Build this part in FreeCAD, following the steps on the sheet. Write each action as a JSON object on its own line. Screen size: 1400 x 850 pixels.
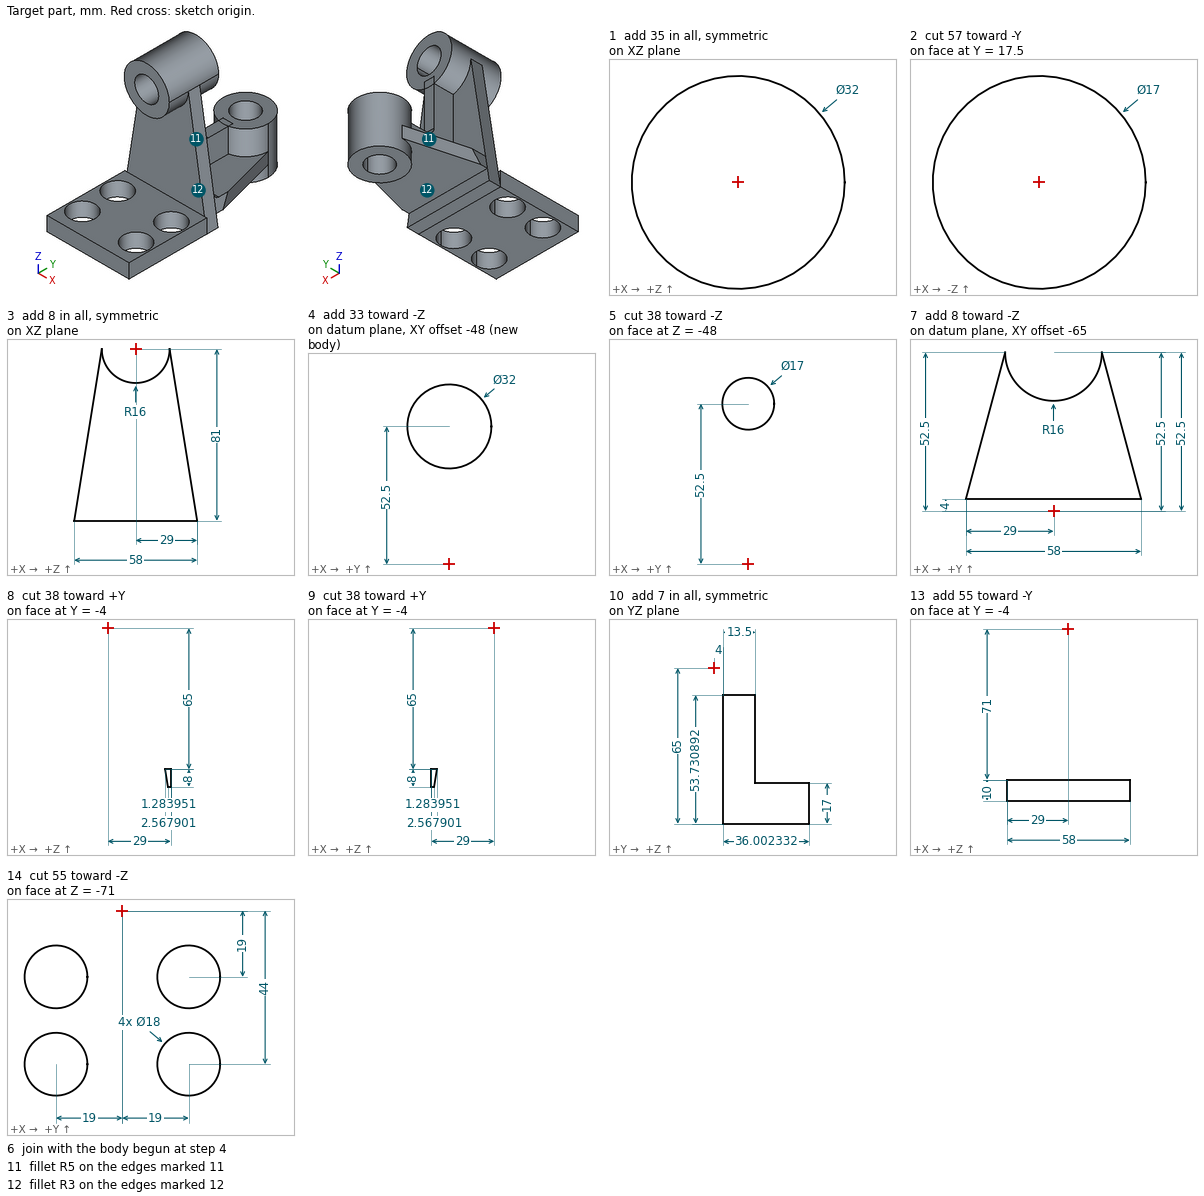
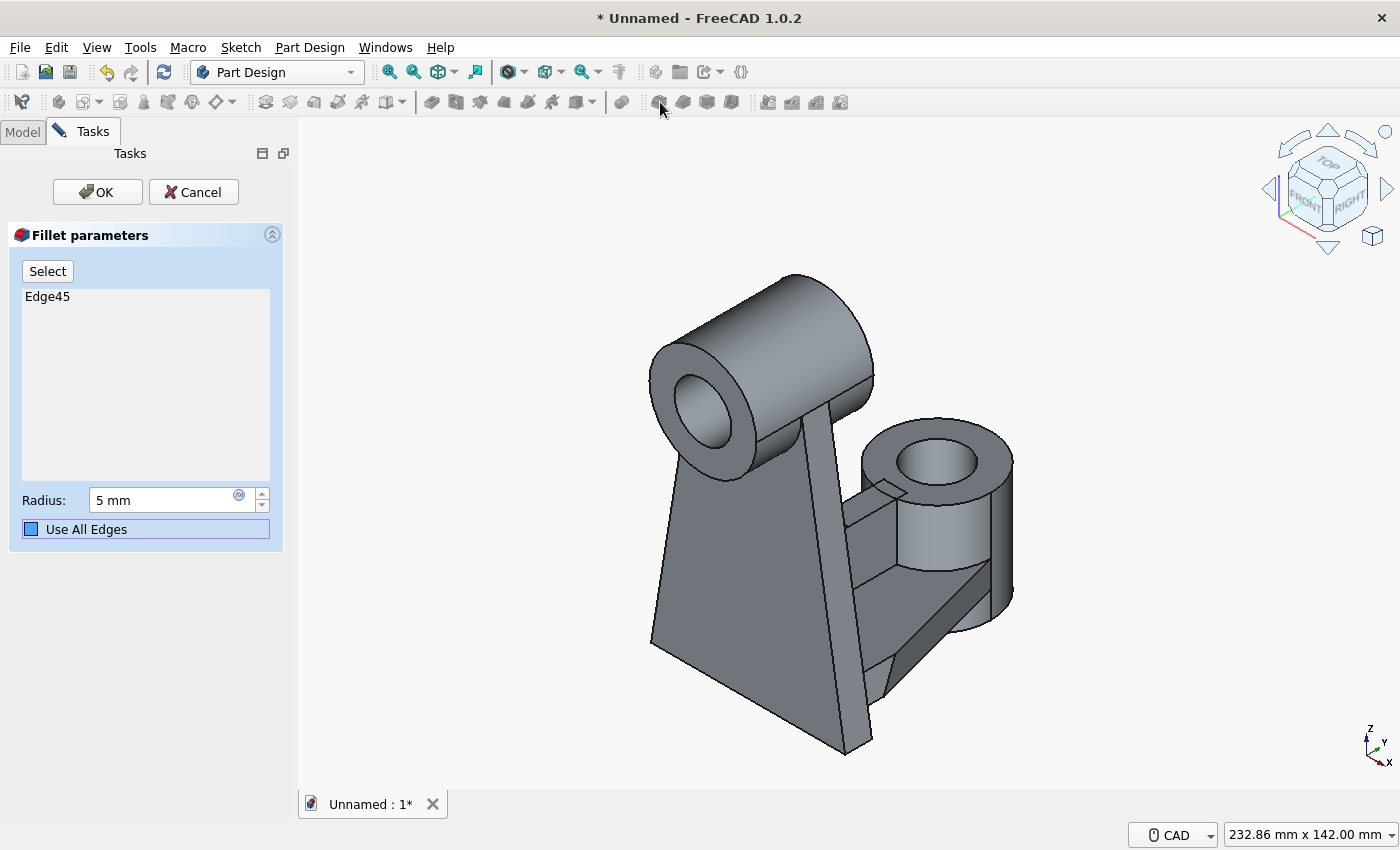
{"action": "left_click", "coordinate": [98, 192]}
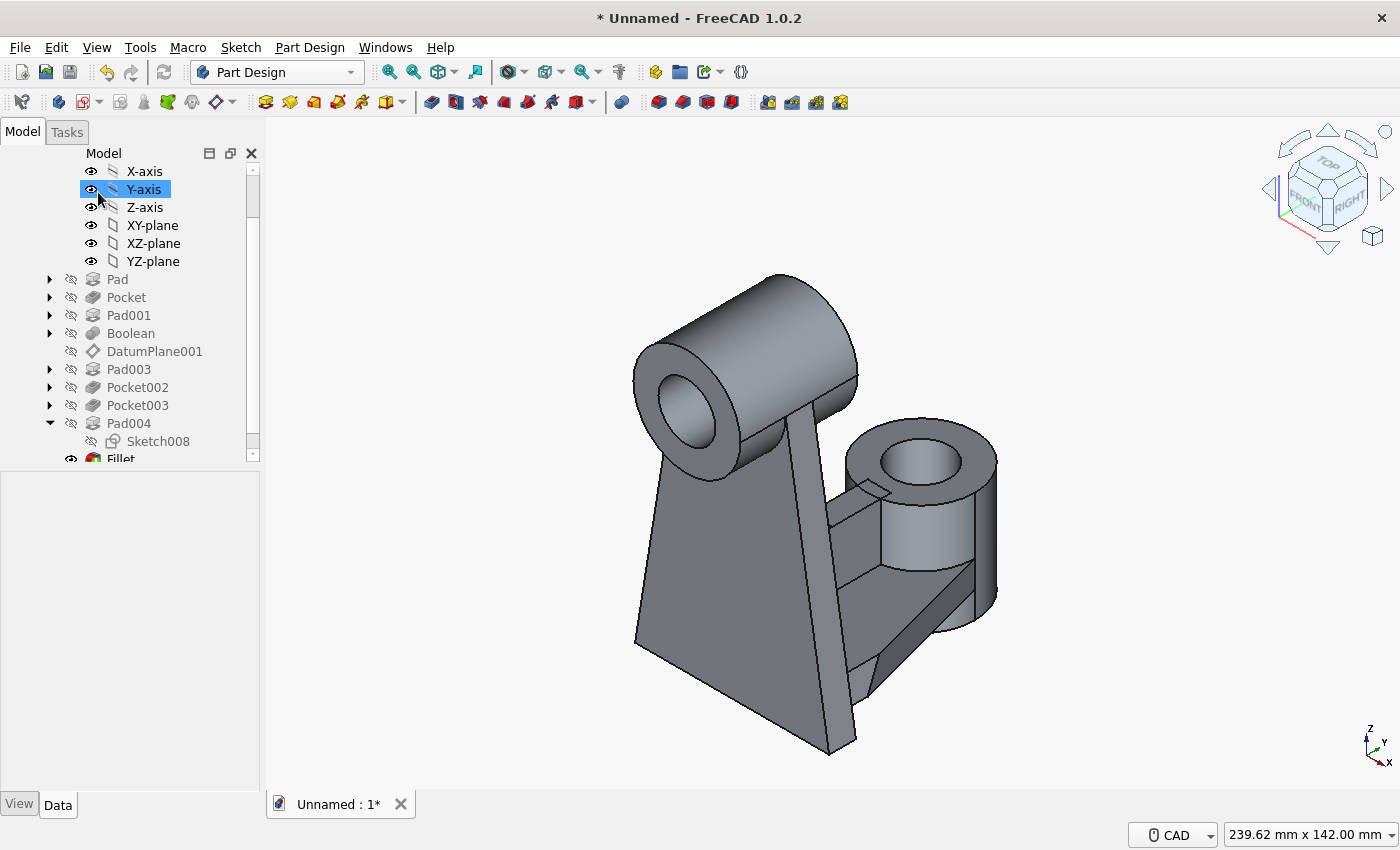
{"action": "key", "text": "2"}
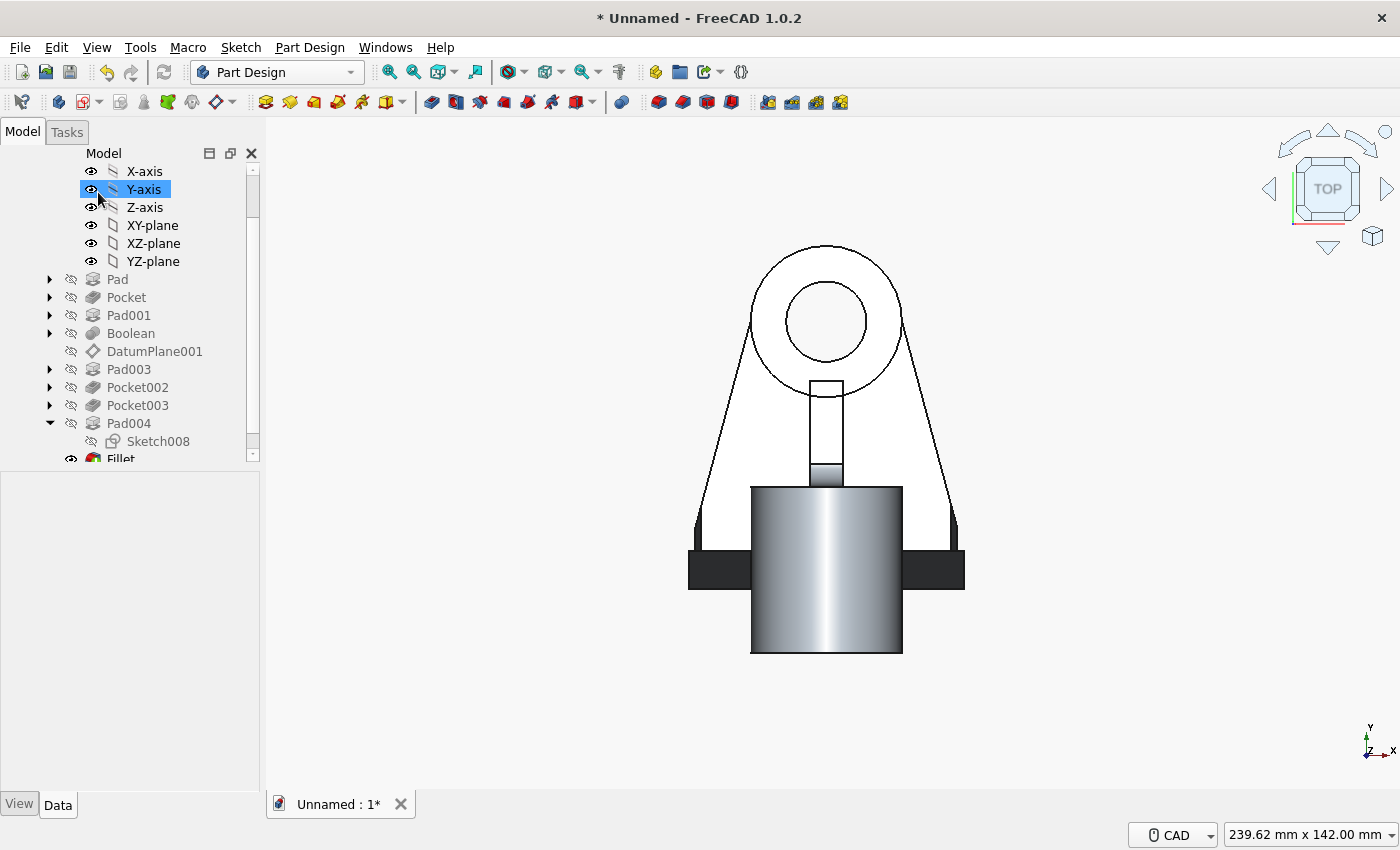
{"action": "key", "text": "0"}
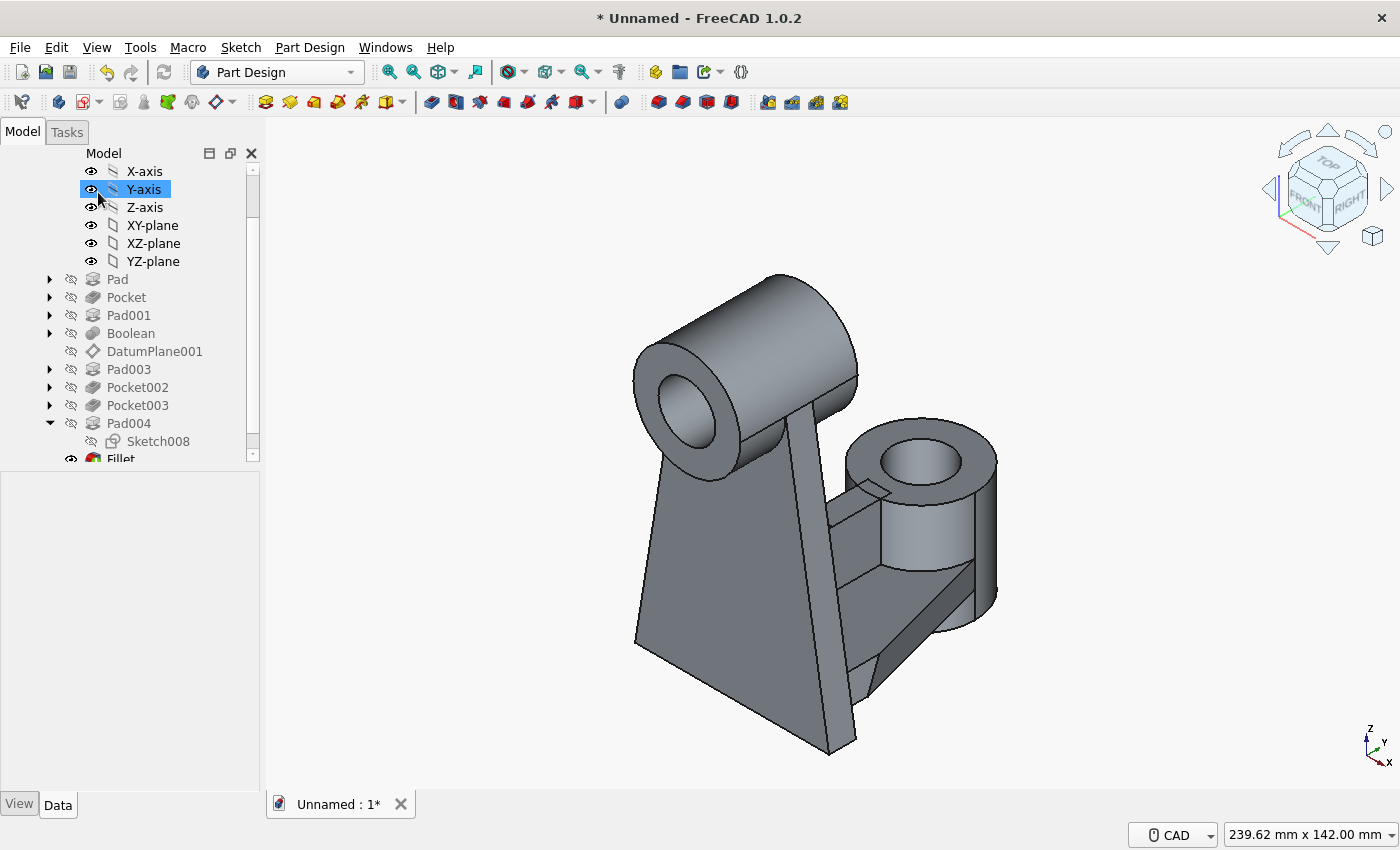
{"action": "key", "text": "1"}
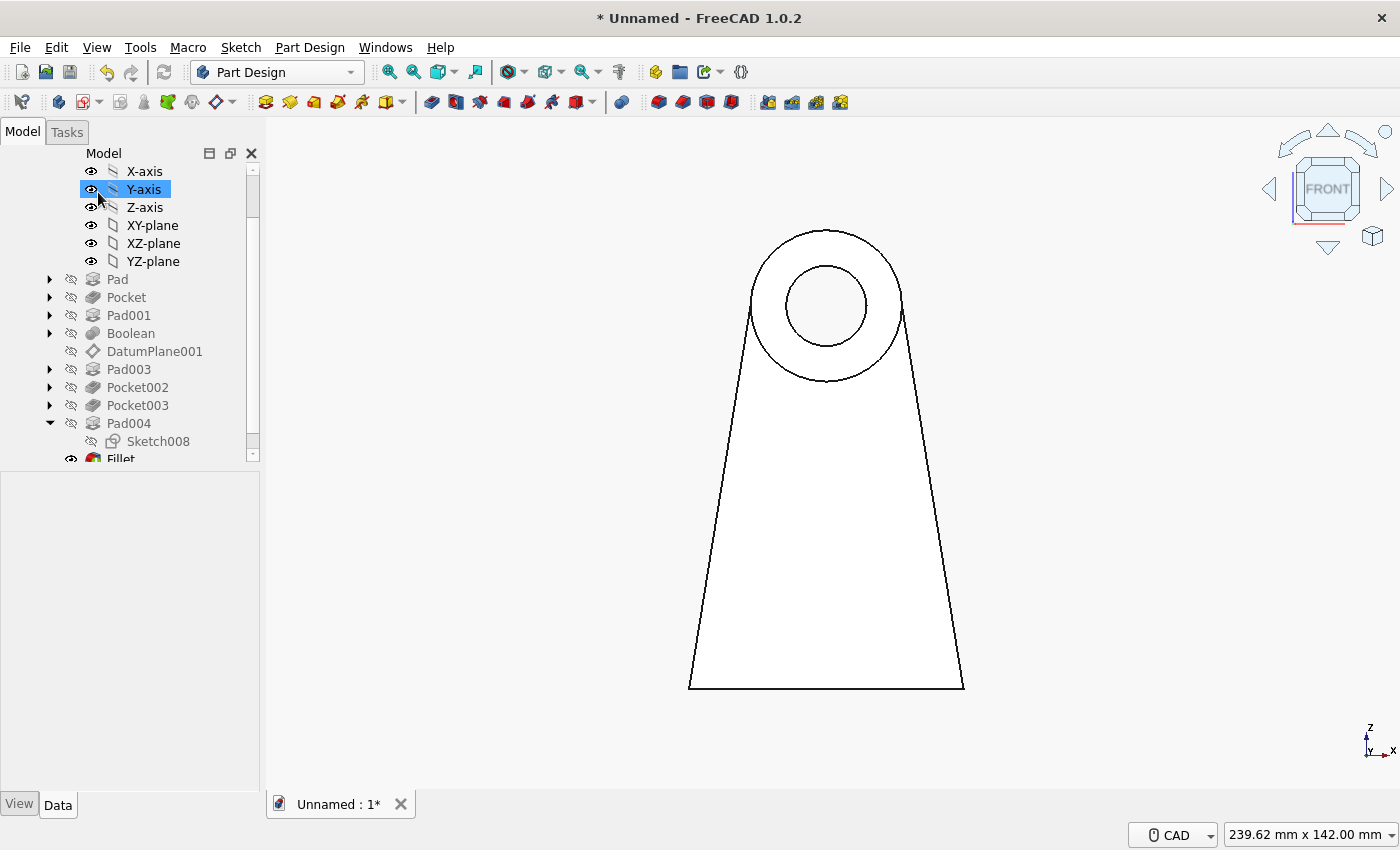
{"action": "key", "text": "3"}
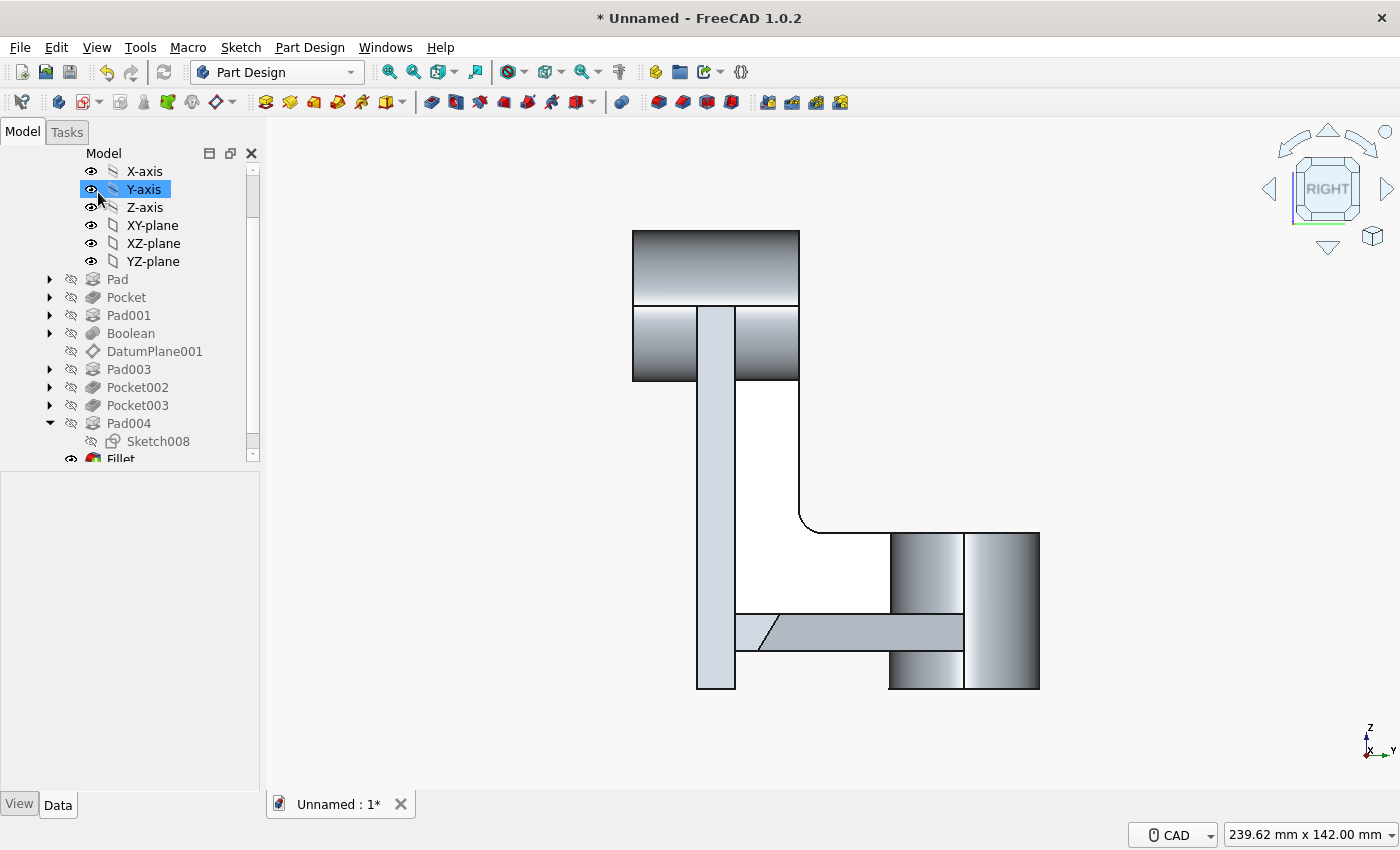
{"action": "key", "text": "5"}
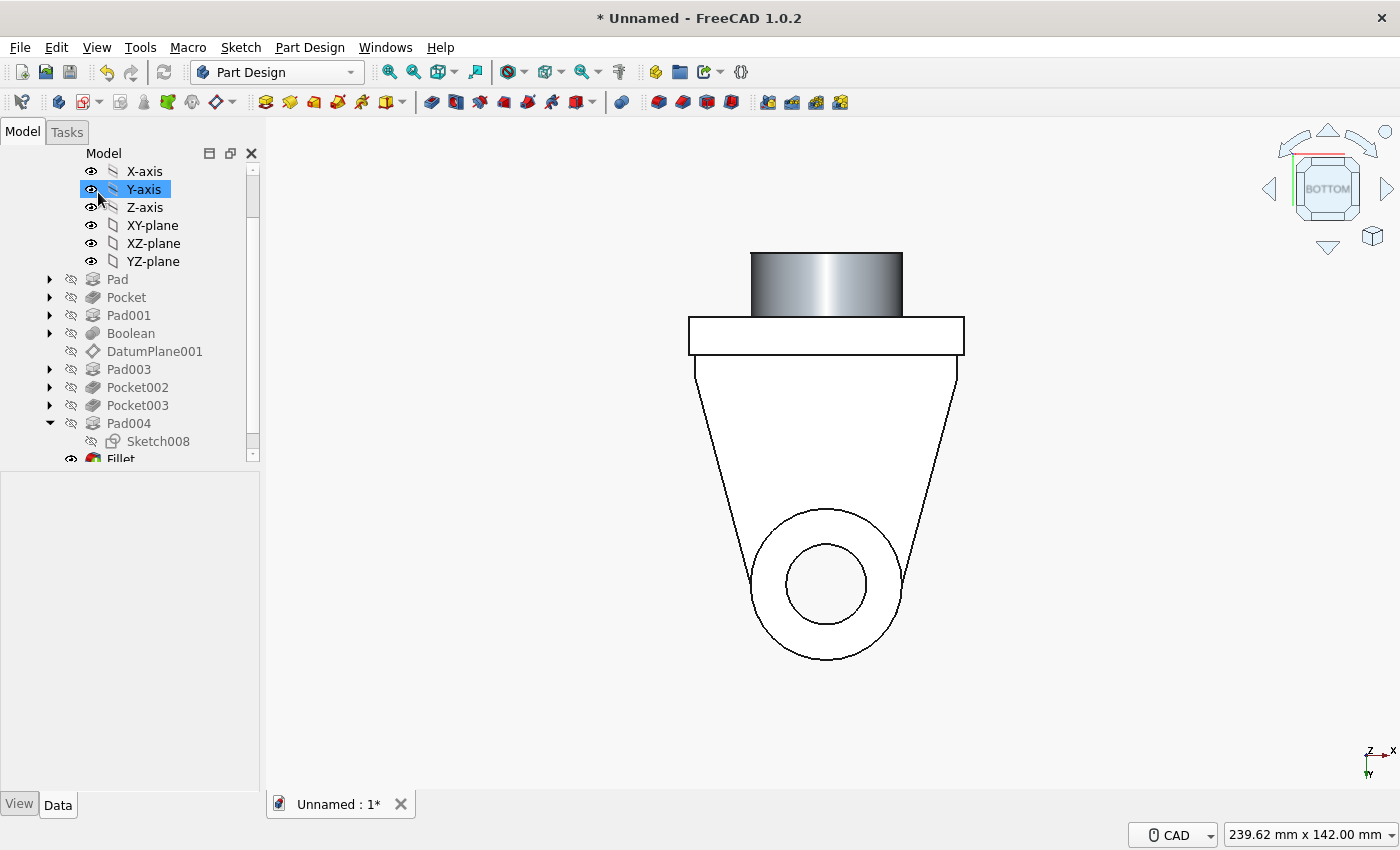
{"action": "key", "text": "4"}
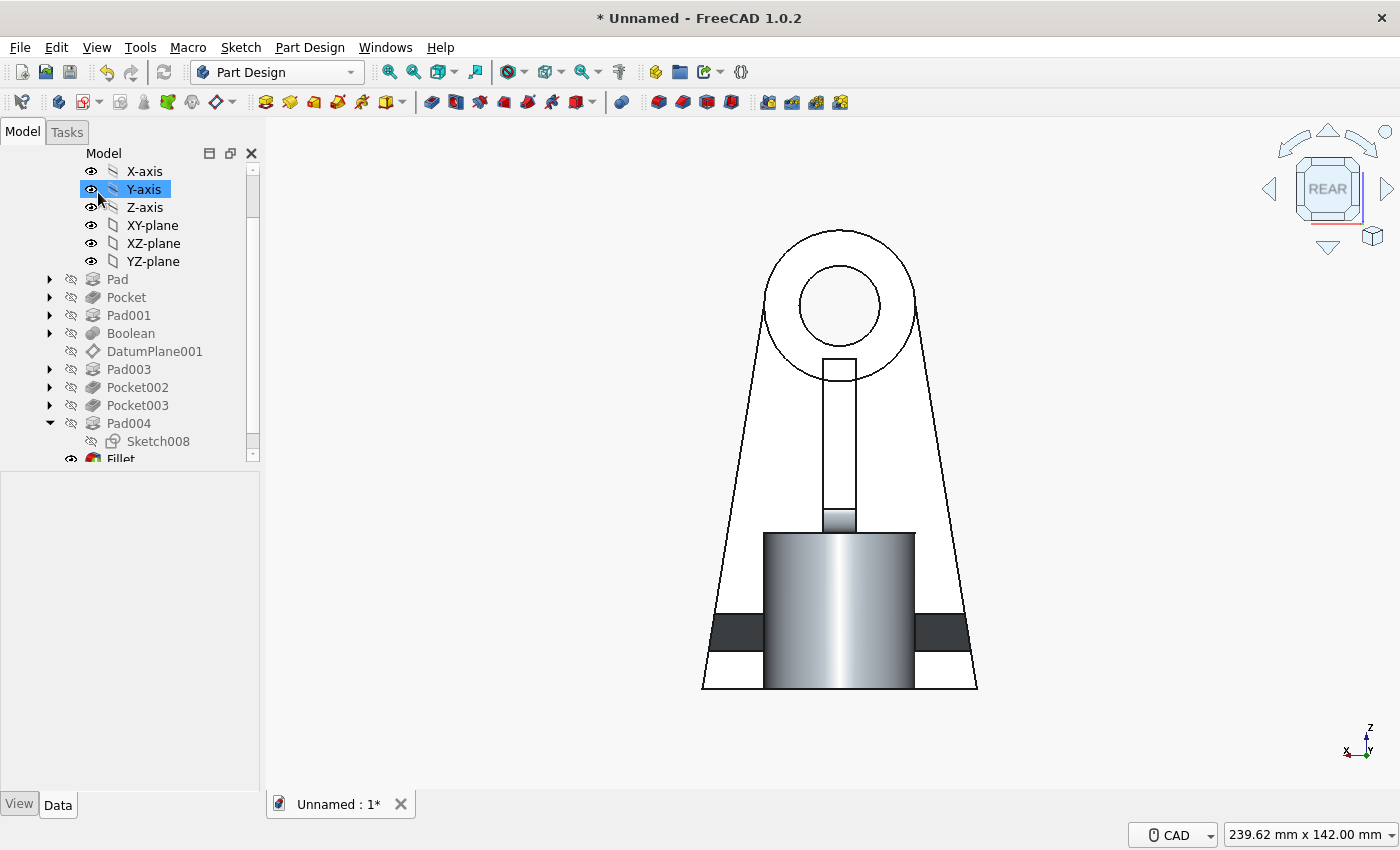
{"action": "key", "text": "6"}